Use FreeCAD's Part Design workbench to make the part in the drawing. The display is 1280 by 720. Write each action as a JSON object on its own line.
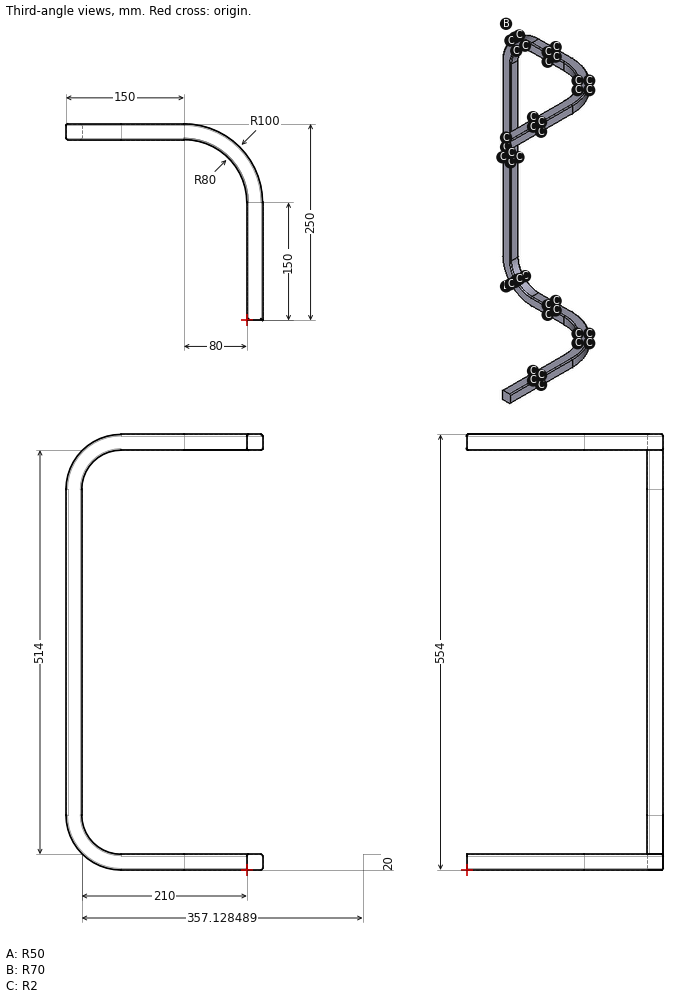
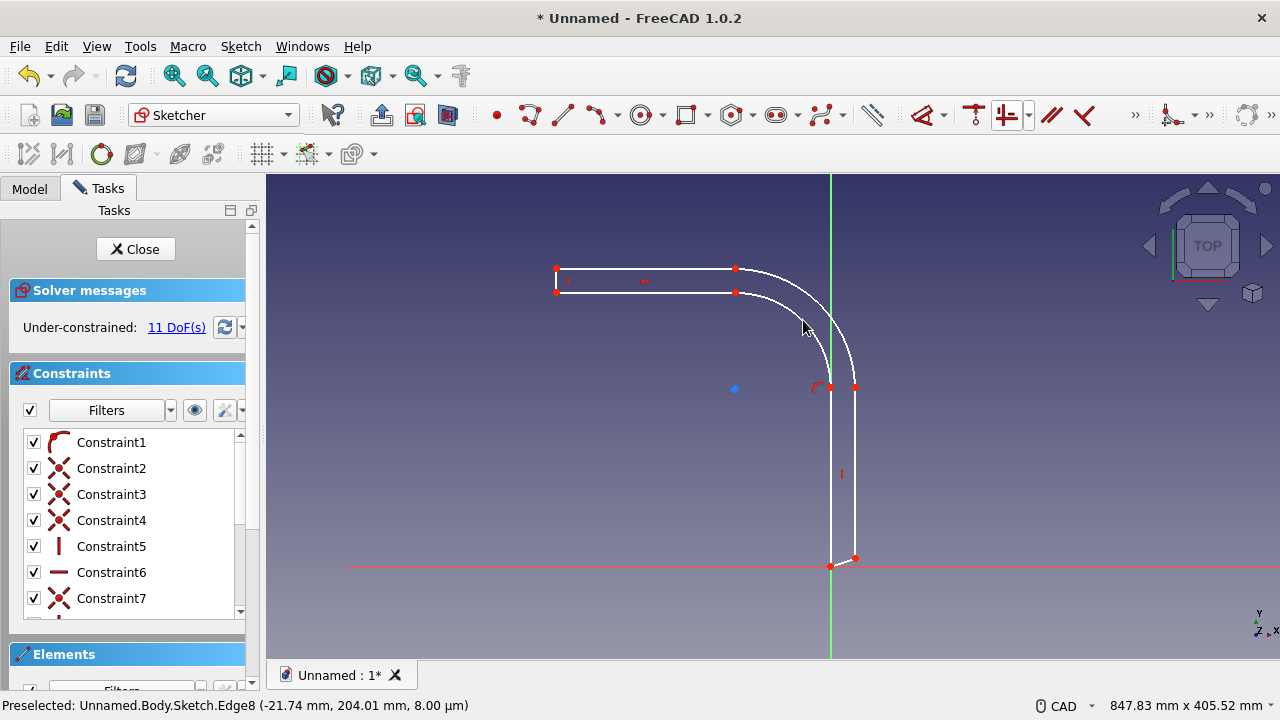
{"action": "scroll", "coordinate": [840, 564], "scroll_direction": "up", "scroll_amount": 2}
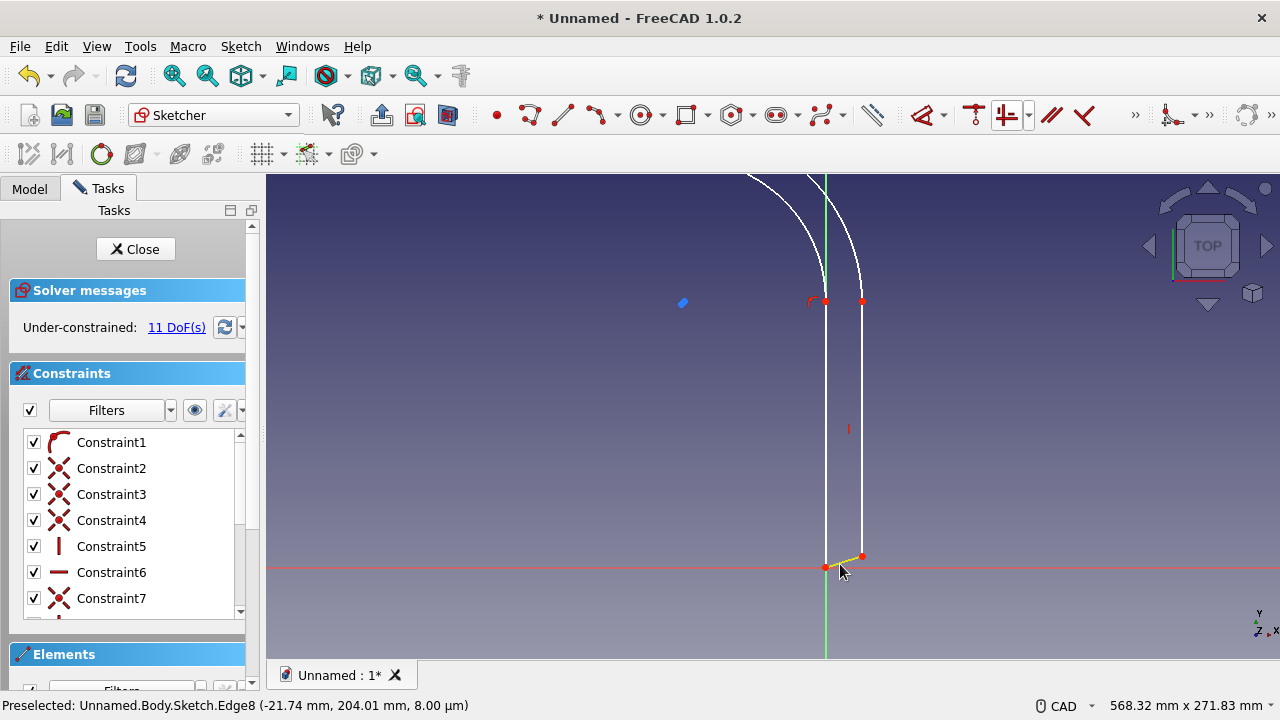
{"action": "left_click", "coordinate": [840, 563]}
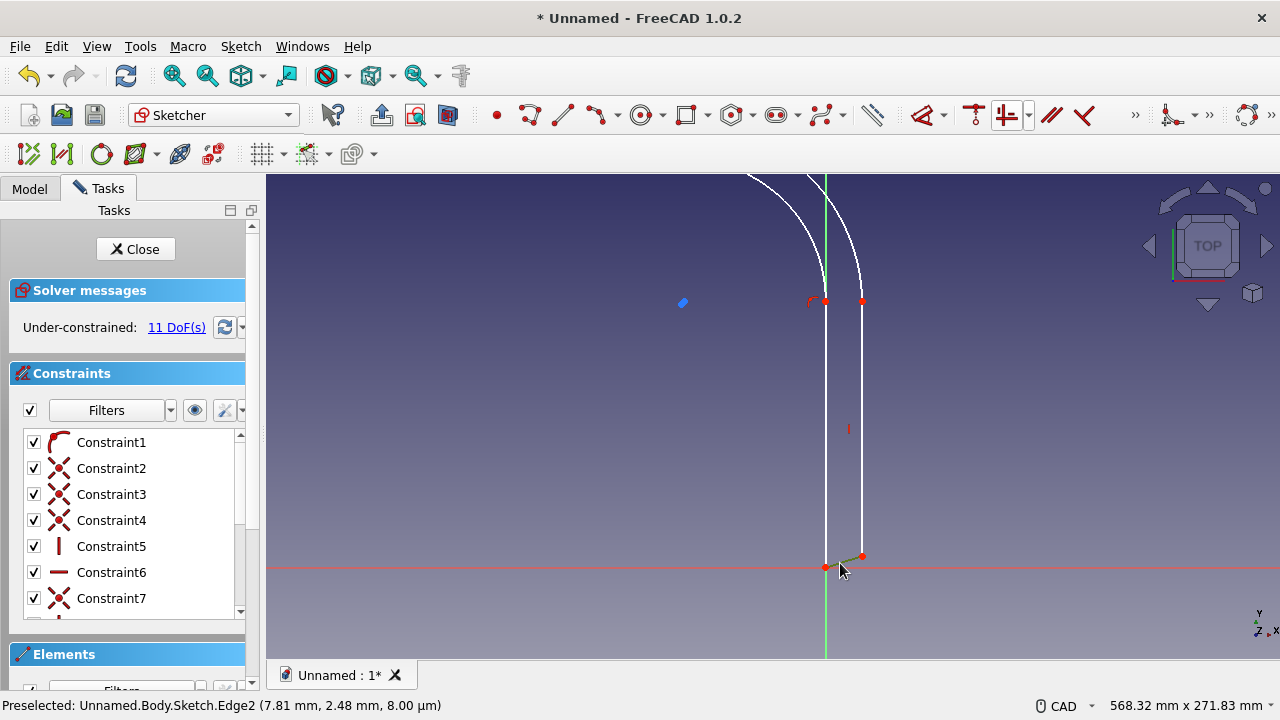
{"action": "left_click", "coordinate": [1028, 116]}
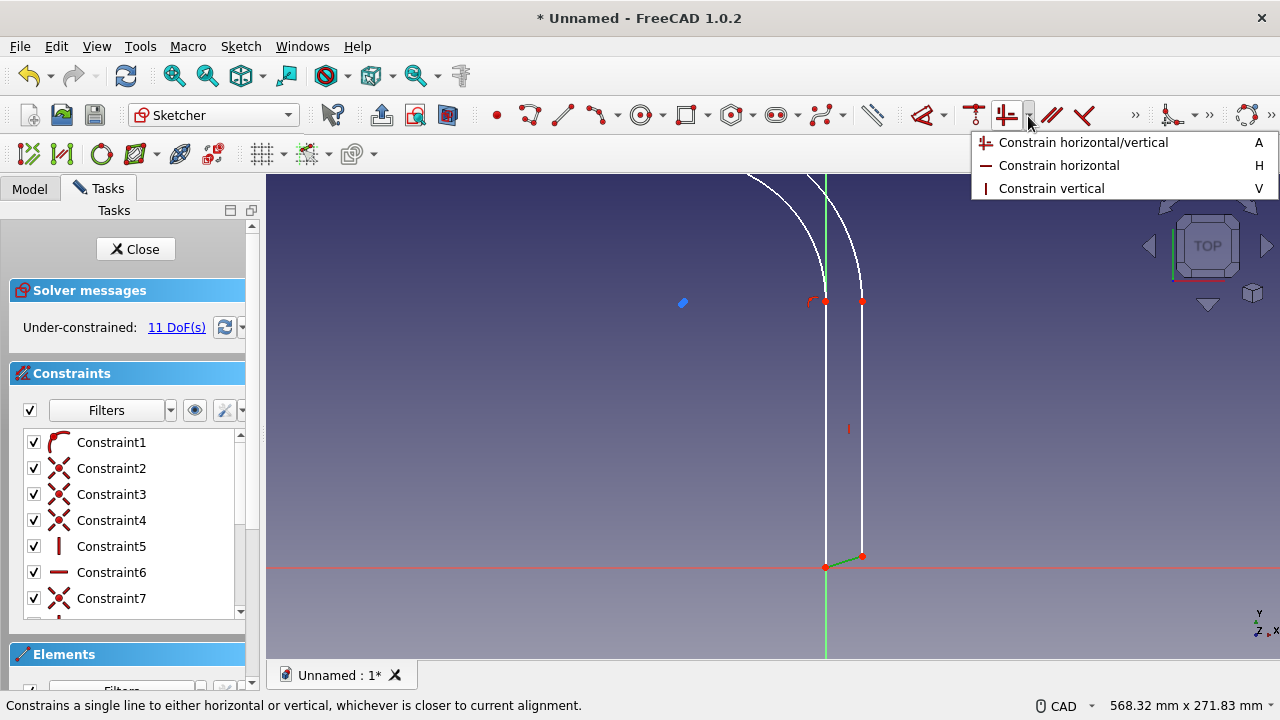
{"action": "left_click", "coordinate": [1125, 166]}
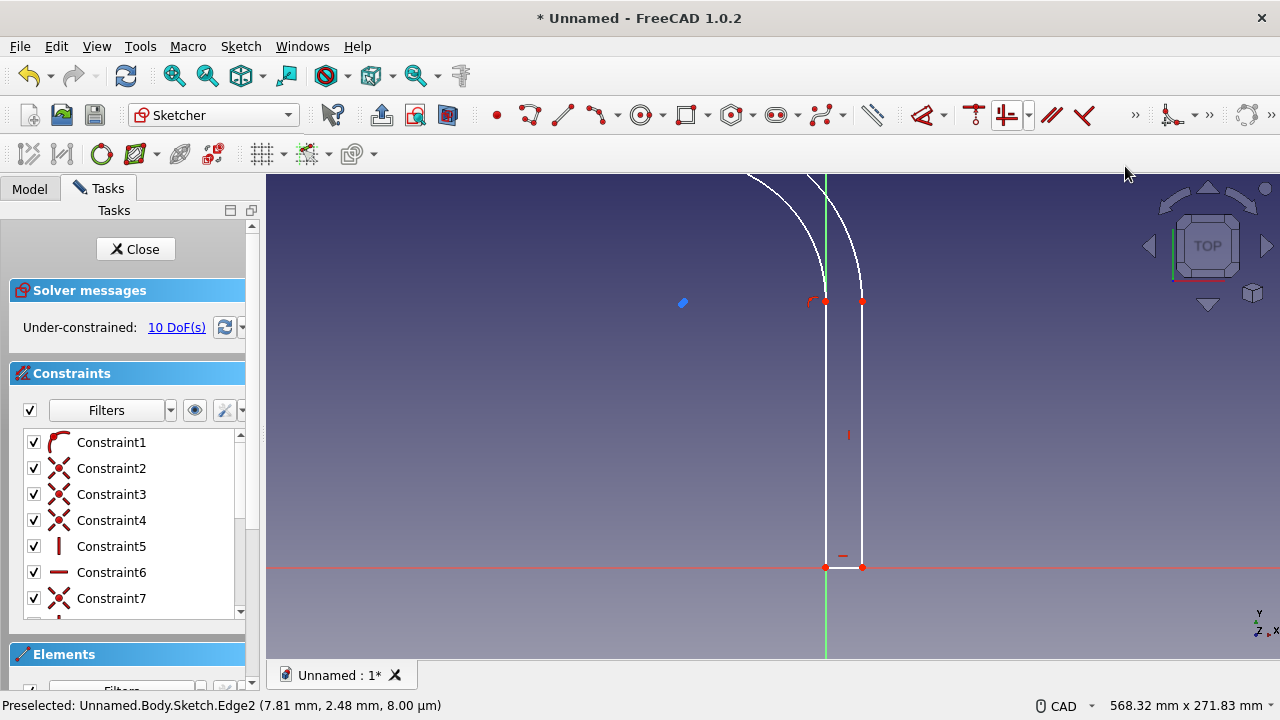
{"action": "left_click", "coordinate": [842, 221]}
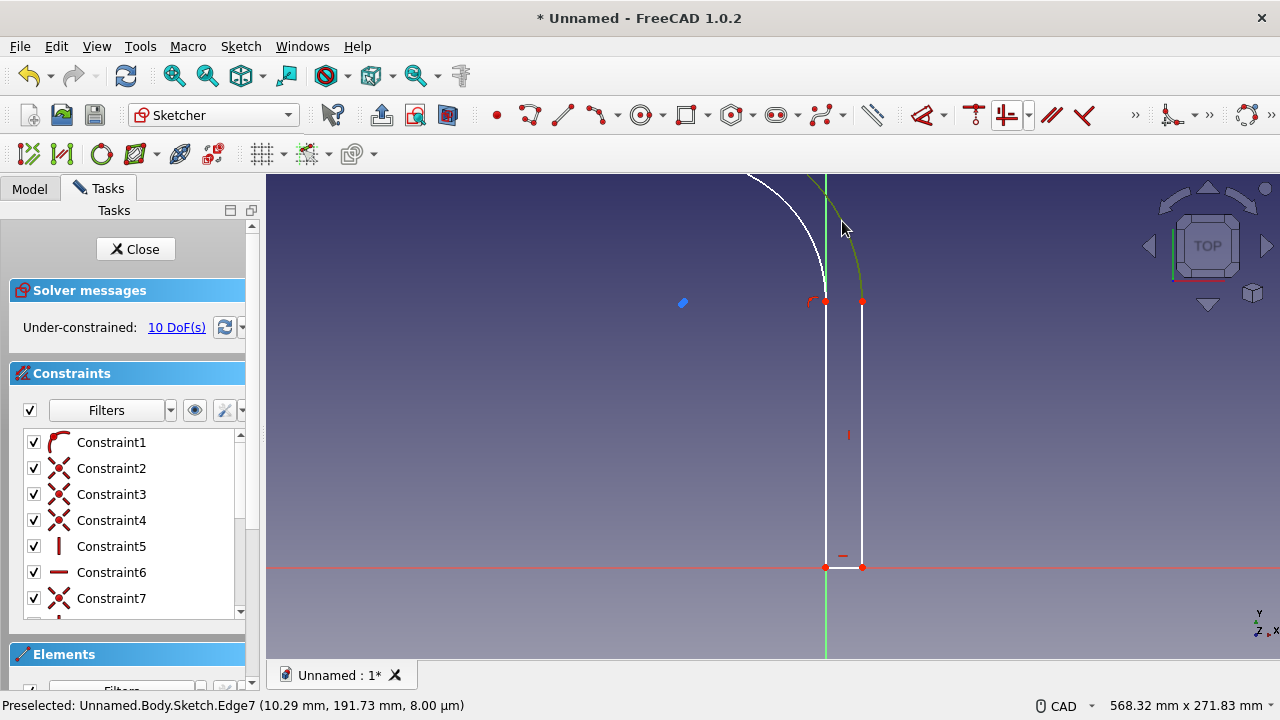
{"action": "left_click", "coordinate": [810, 236]}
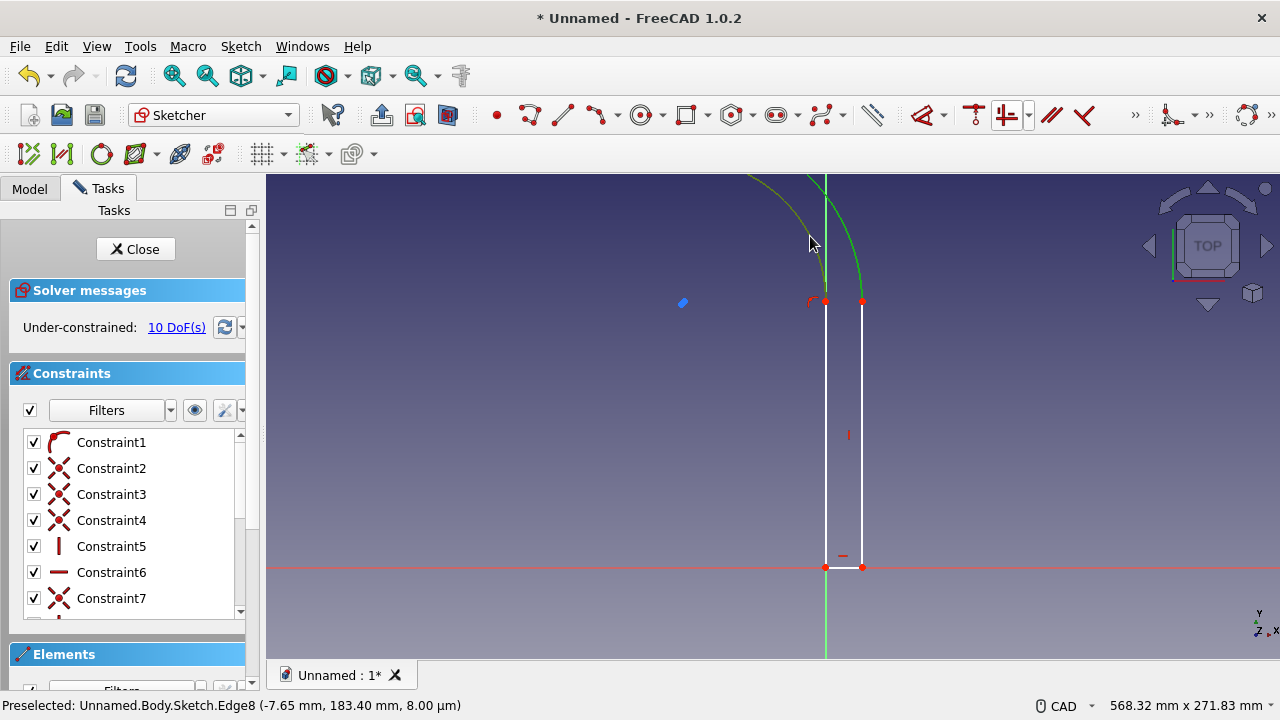
{"action": "left_click", "coordinate": [974, 116]}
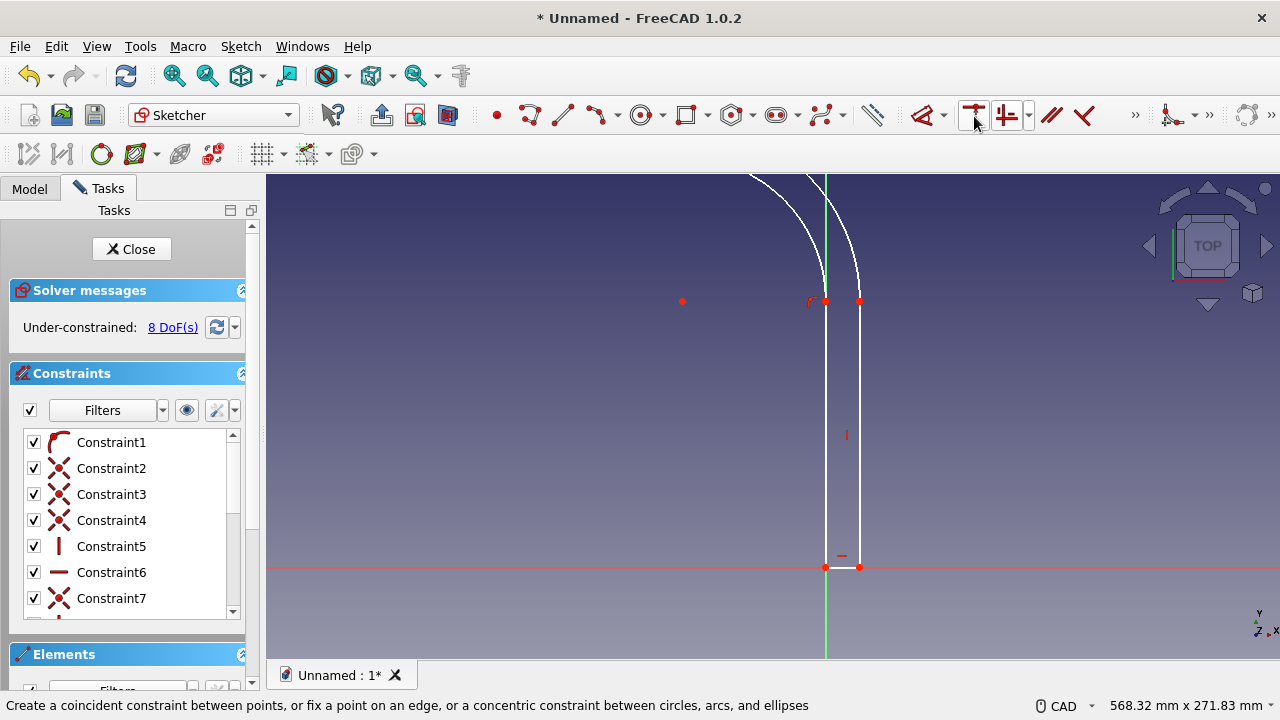
{"action": "left_click", "coordinate": [841, 221]}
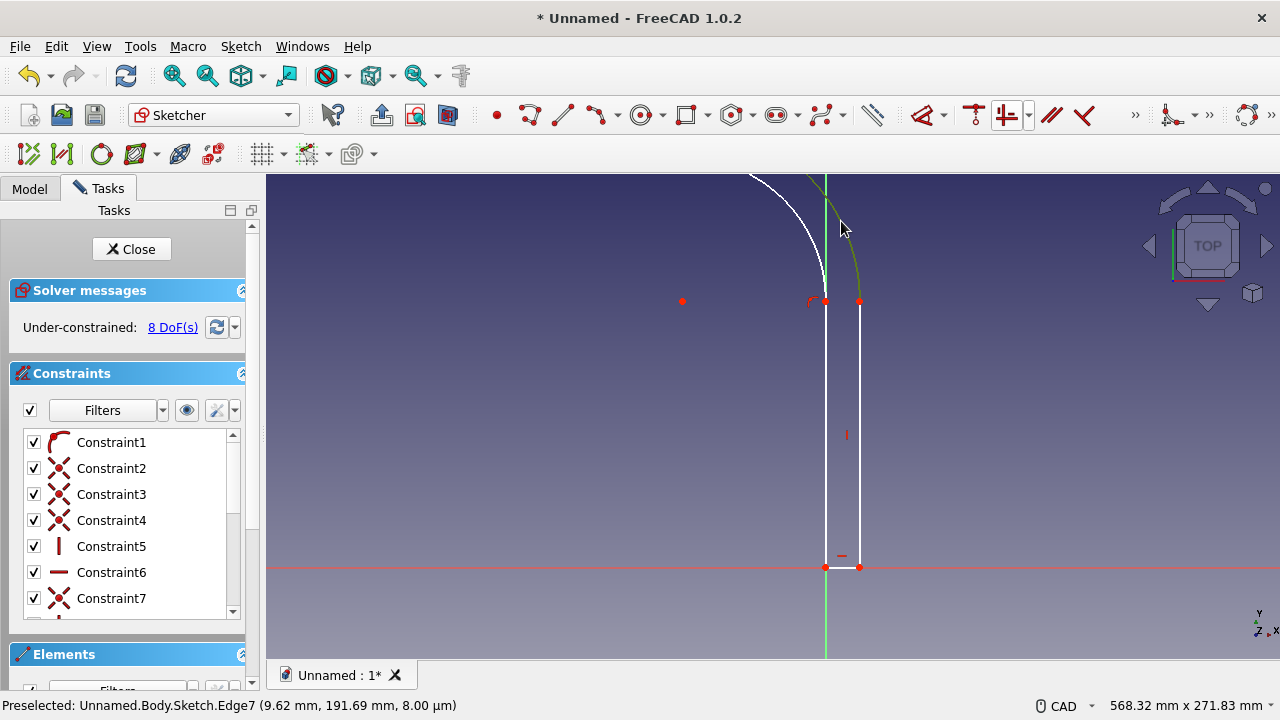
{"action": "left_click", "coordinate": [944, 116]}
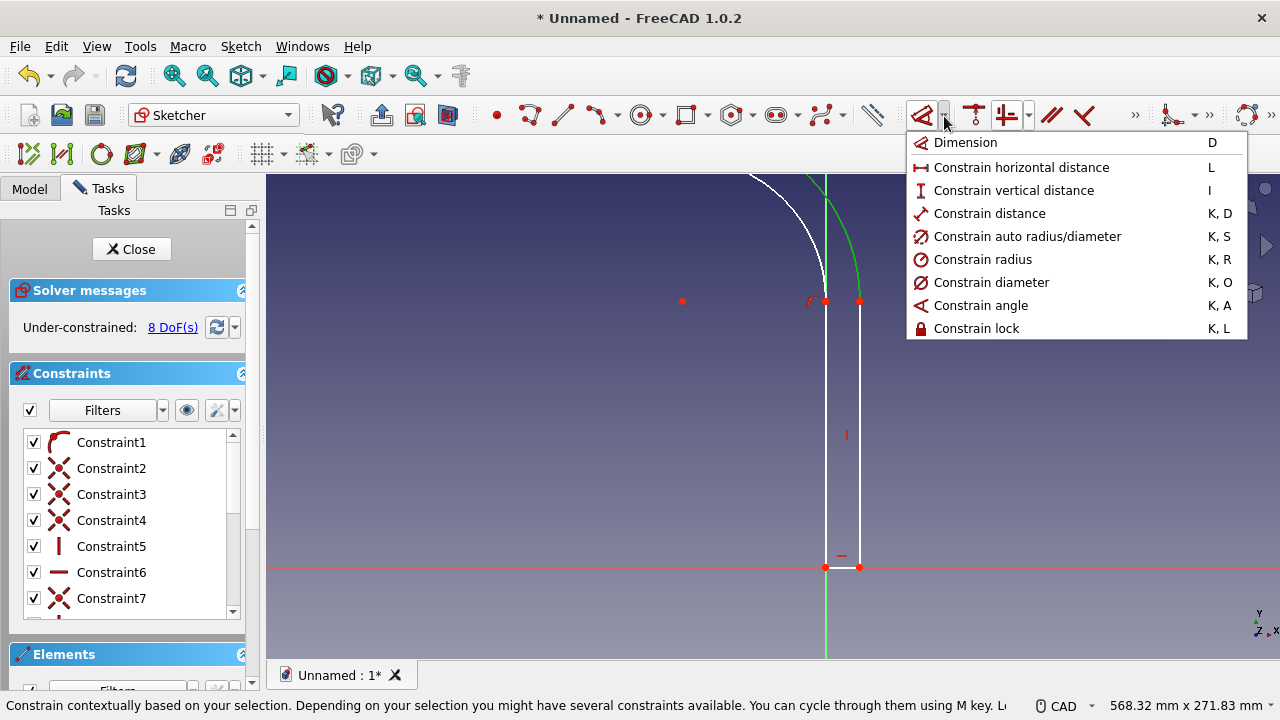
{"action": "left_click", "coordinate": [1077, 260]}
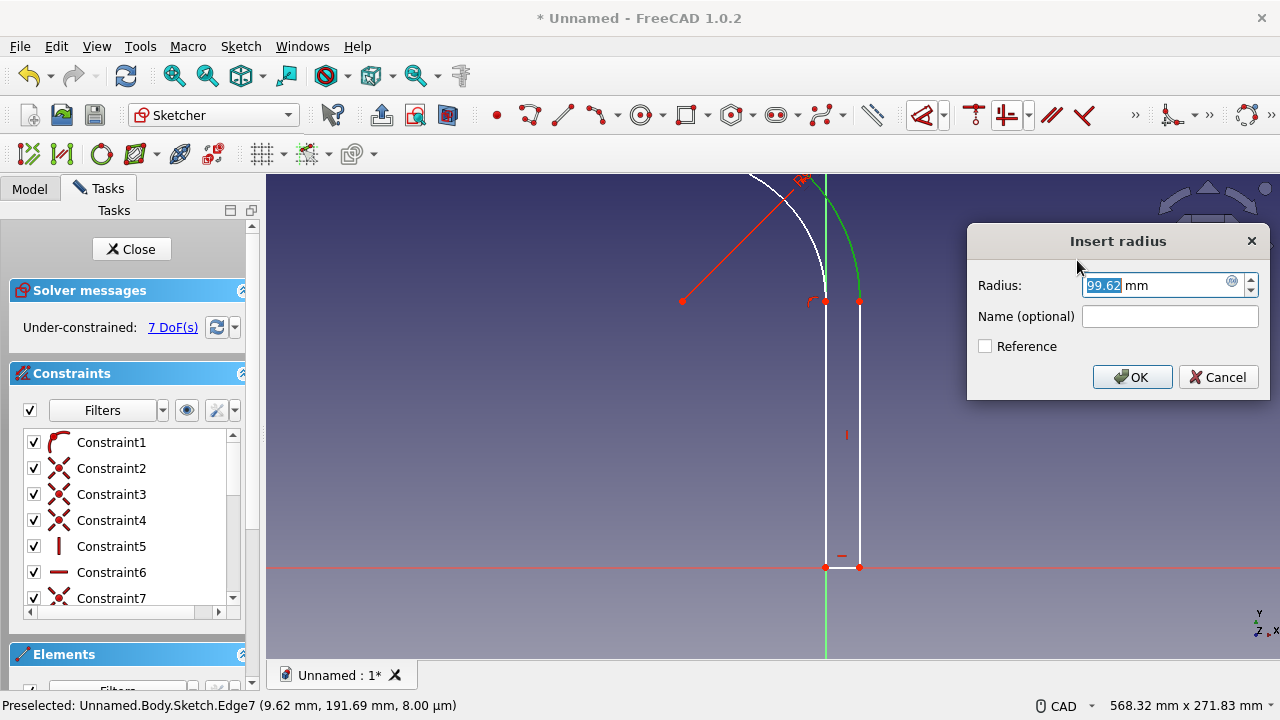
{"action": "type", "text": "100"}
{"action": "key", "text": "Return"}